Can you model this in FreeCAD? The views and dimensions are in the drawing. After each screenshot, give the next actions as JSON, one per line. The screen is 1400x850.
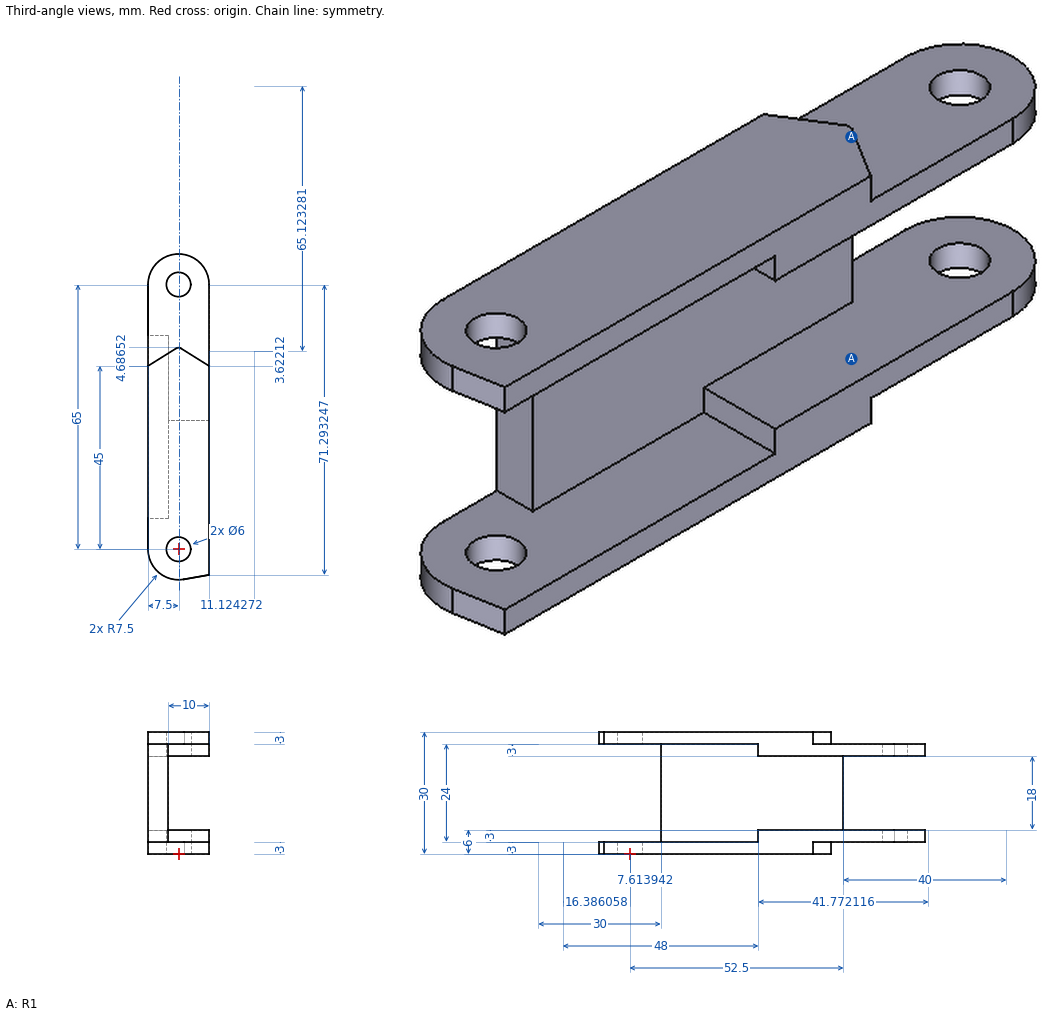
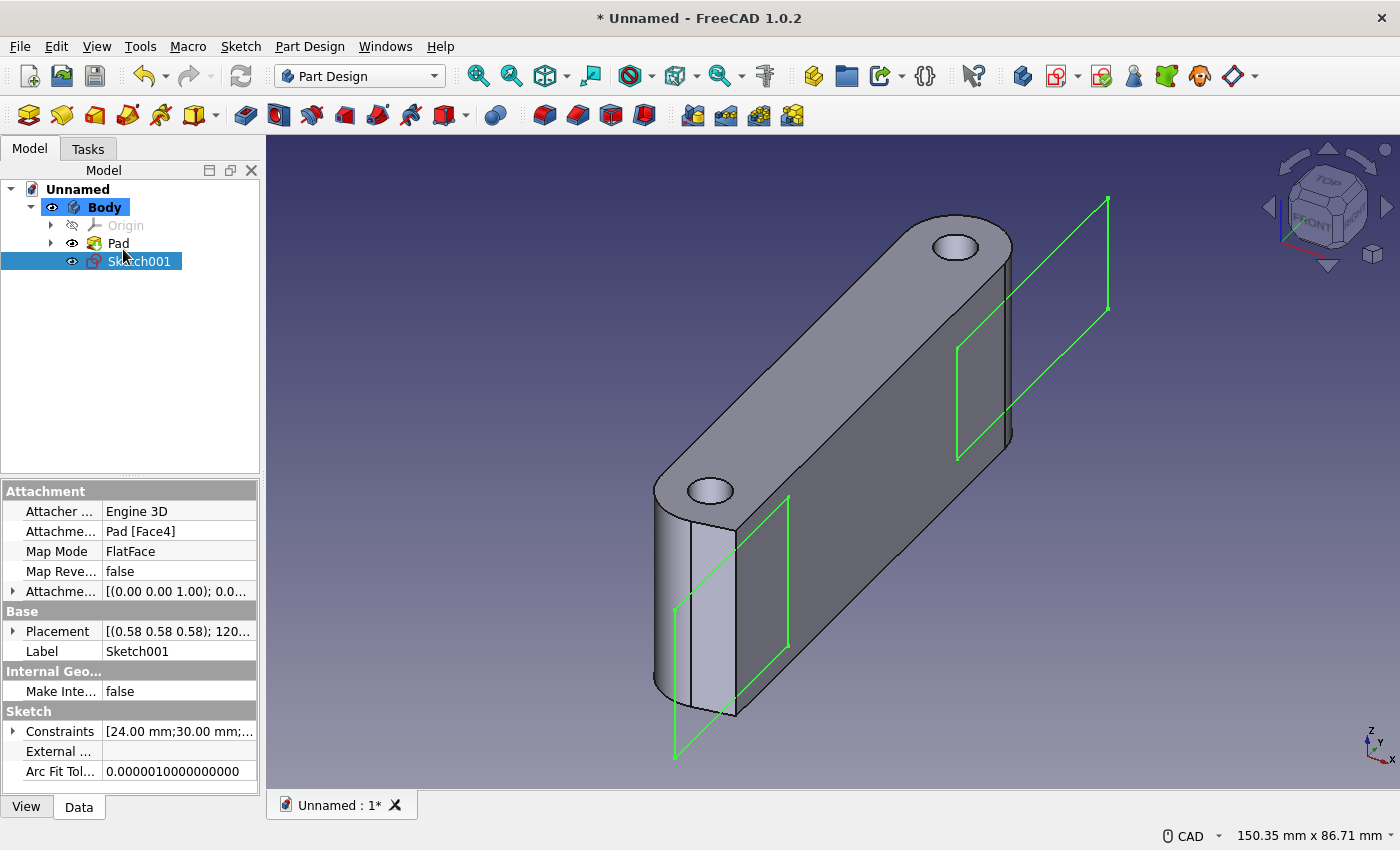
{"action": "left_click", "coordinate": [246, 116]}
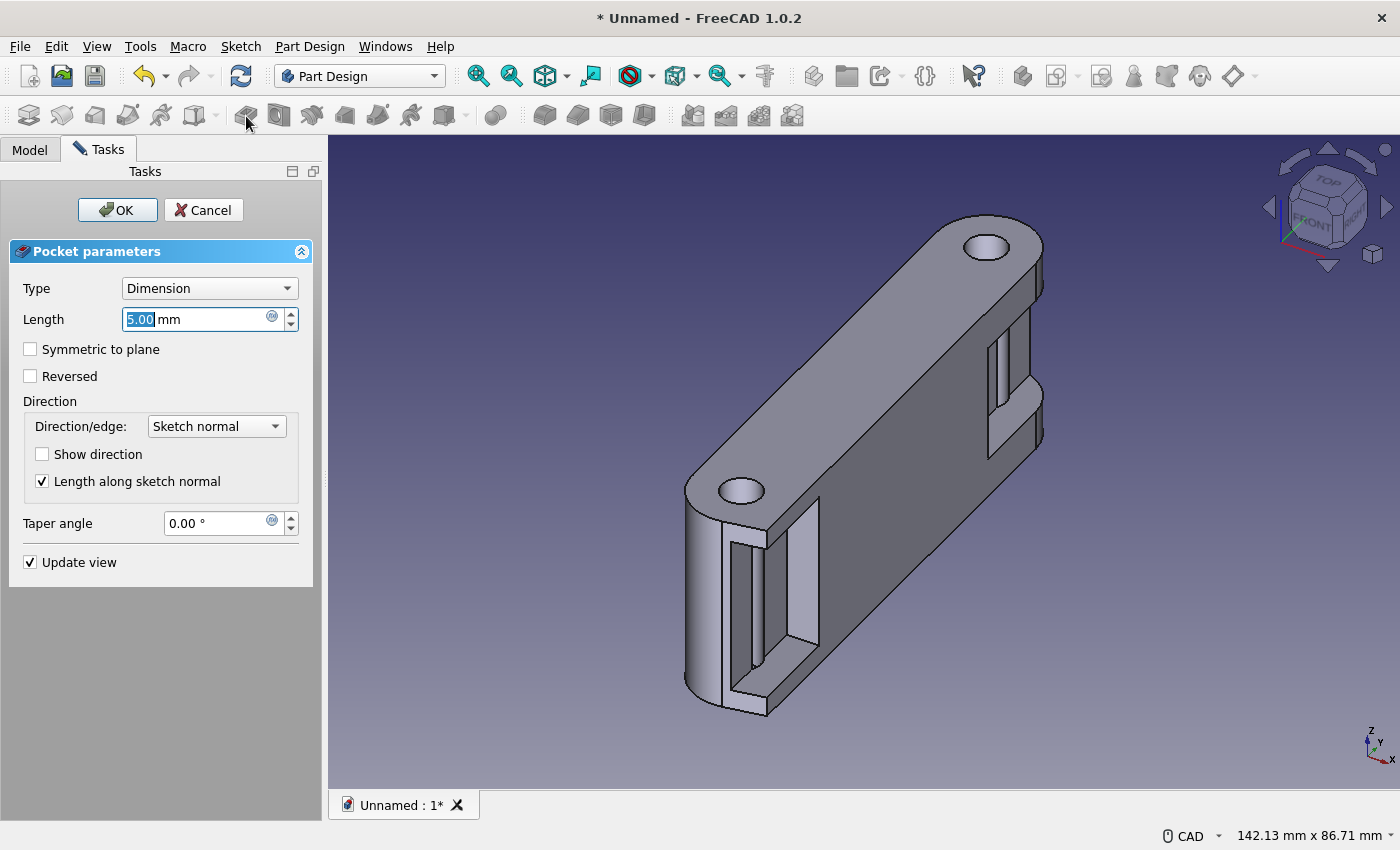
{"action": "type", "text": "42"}
{"action": "key", "text": "Tab"}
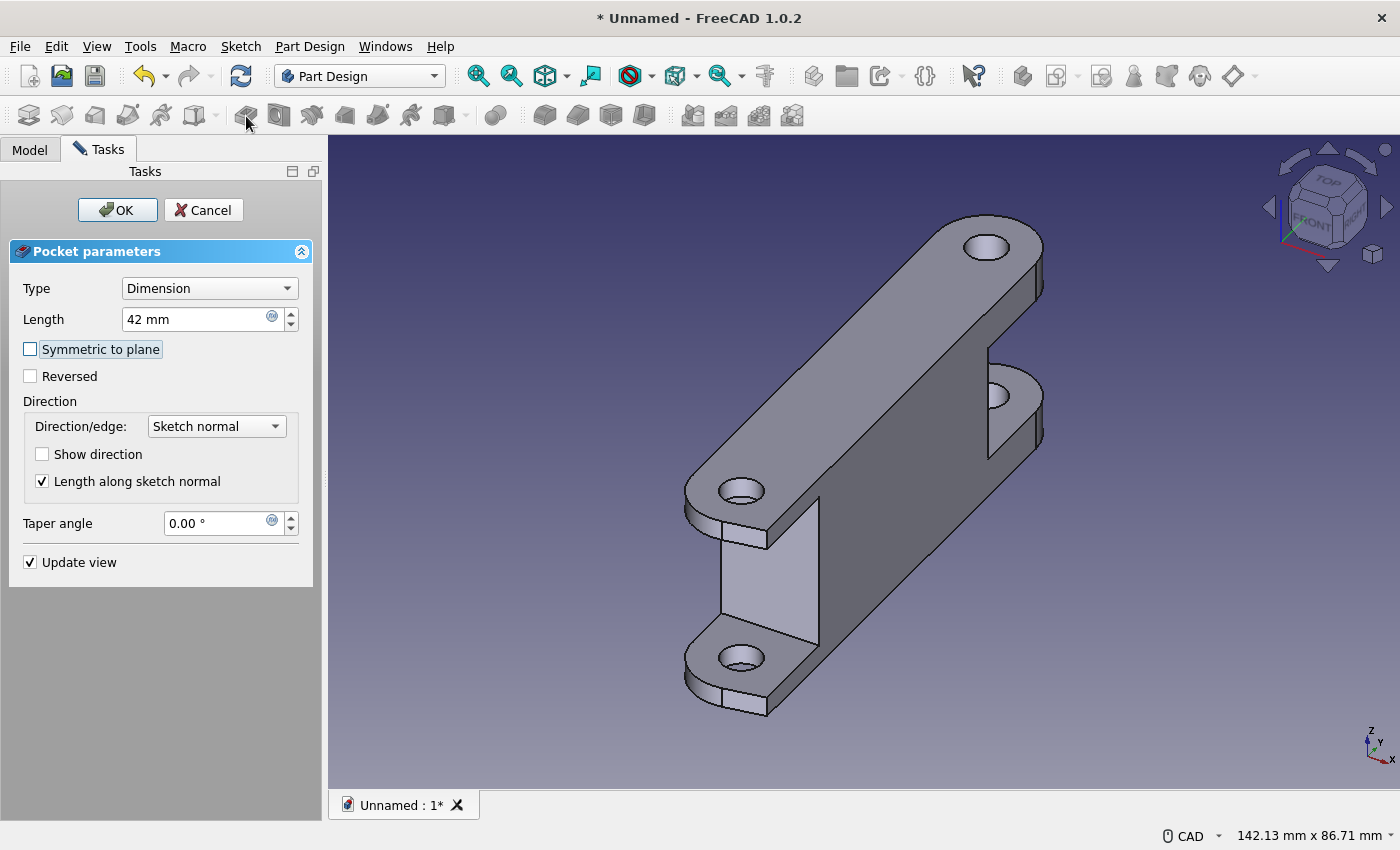
{"action": "left_click", "coordinate": [118, 210]}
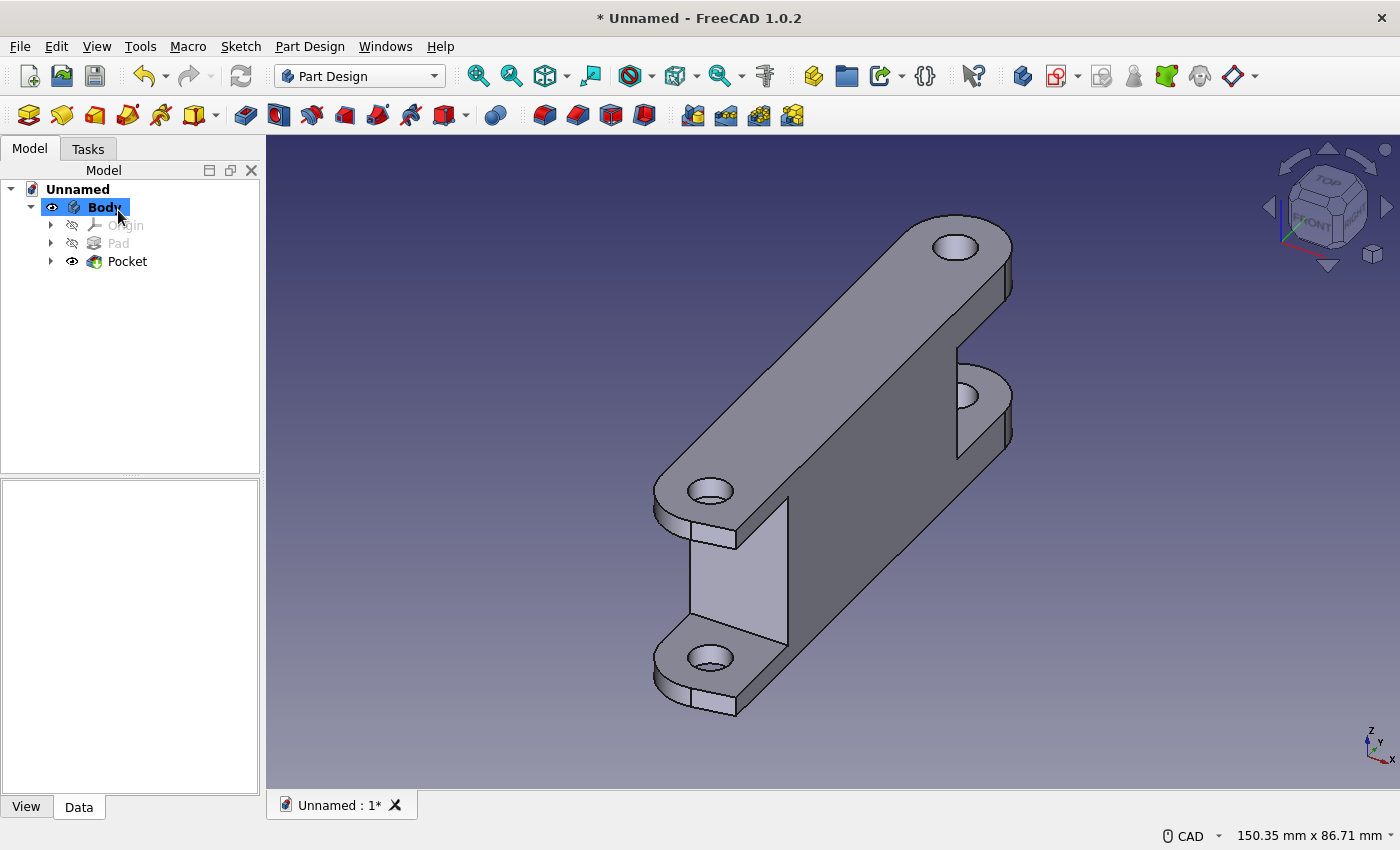
{"action": "left_click", "coordinate": [876, 325]}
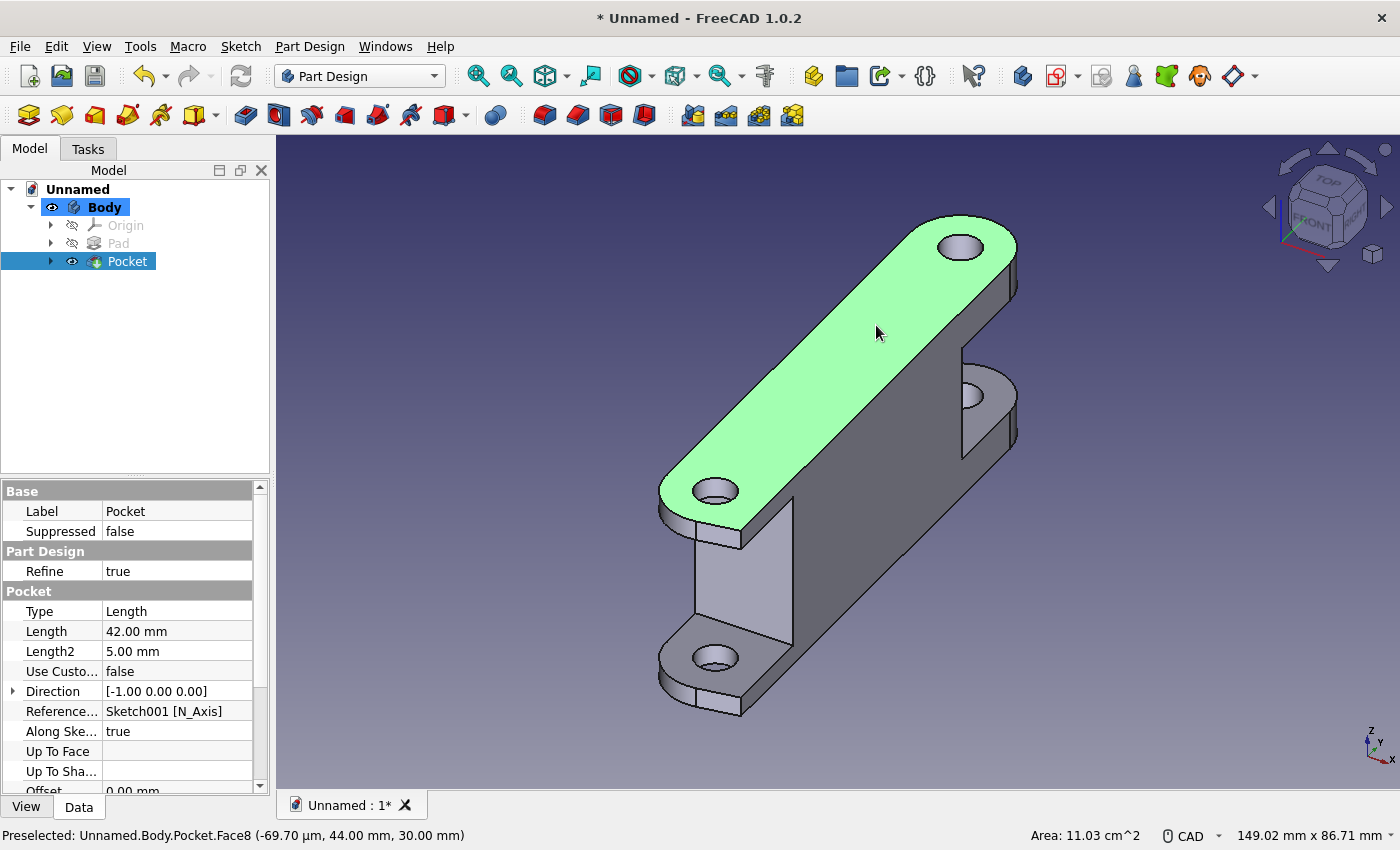
{"action": "left_click", "coordinate": [1056, 76]}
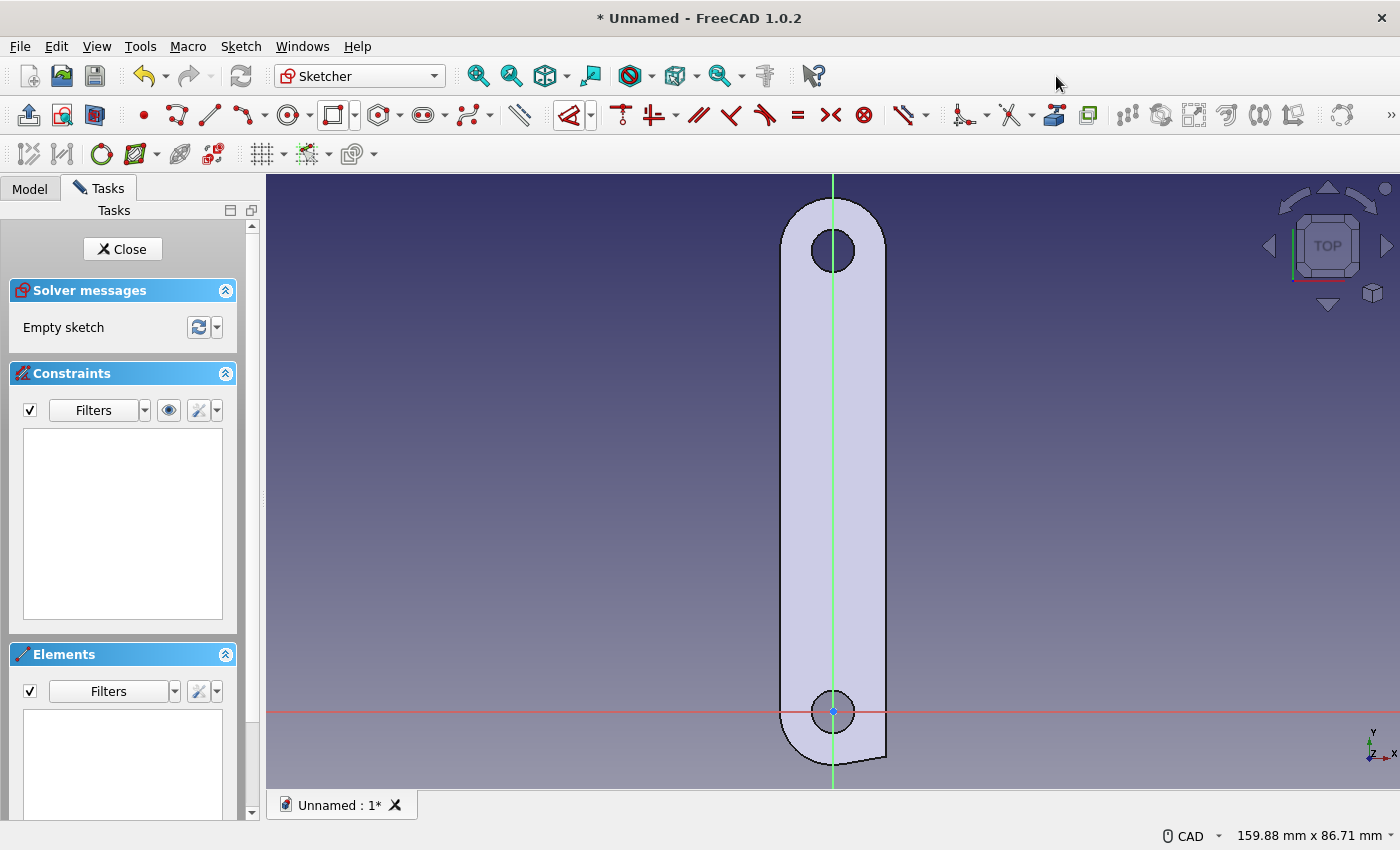
{"action": "scroll", "coordinate": [709, 623], "scroll_direction": "down", "scroll_amount": 4}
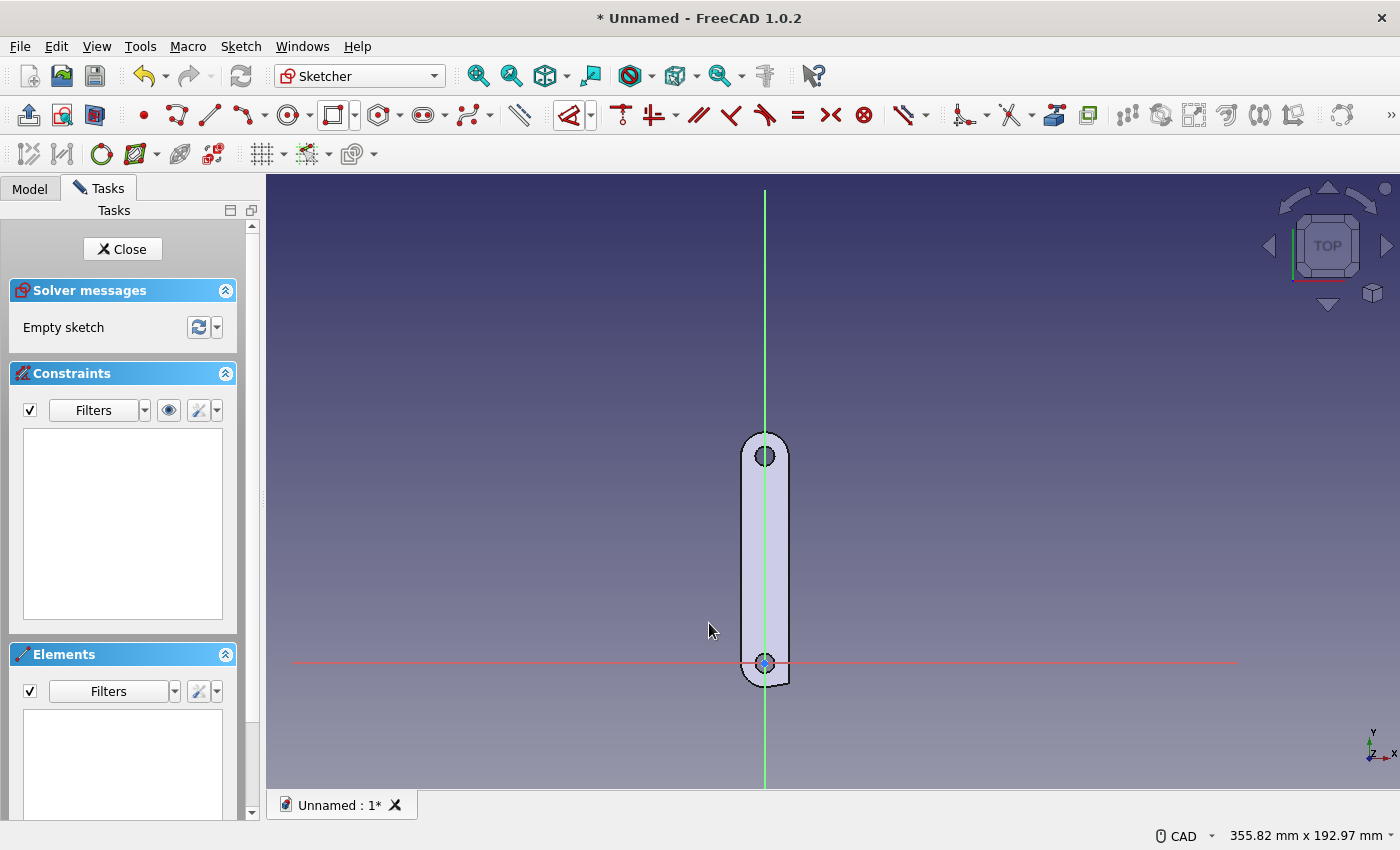
{"action": "key", "text": "g m"}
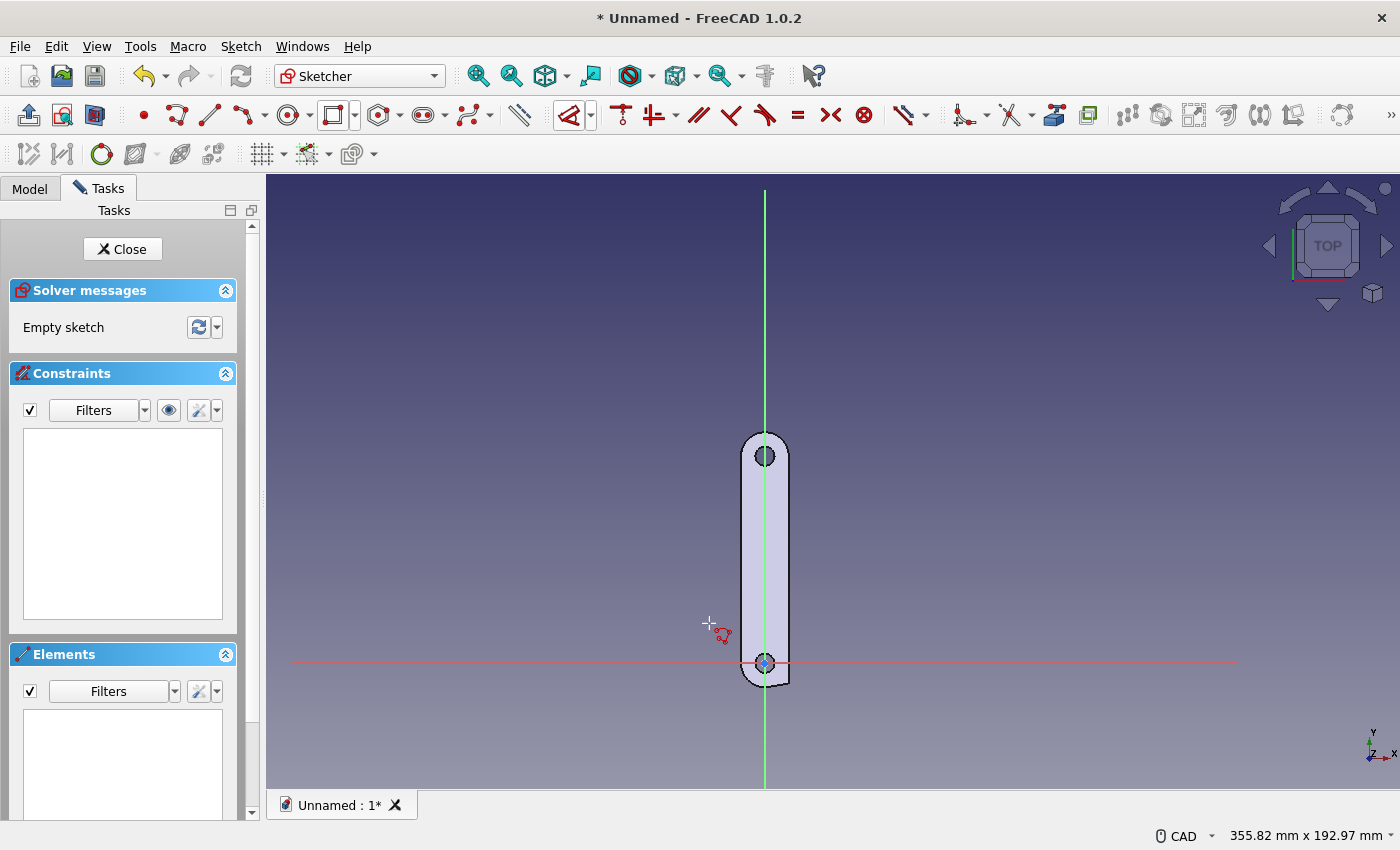
{"action": "left_click", "coordinate": [741, 520]}
{"action": "left_click", "coordinate": [765, 505]}
{"action": "left_click", "coordinate": [789, 520]}